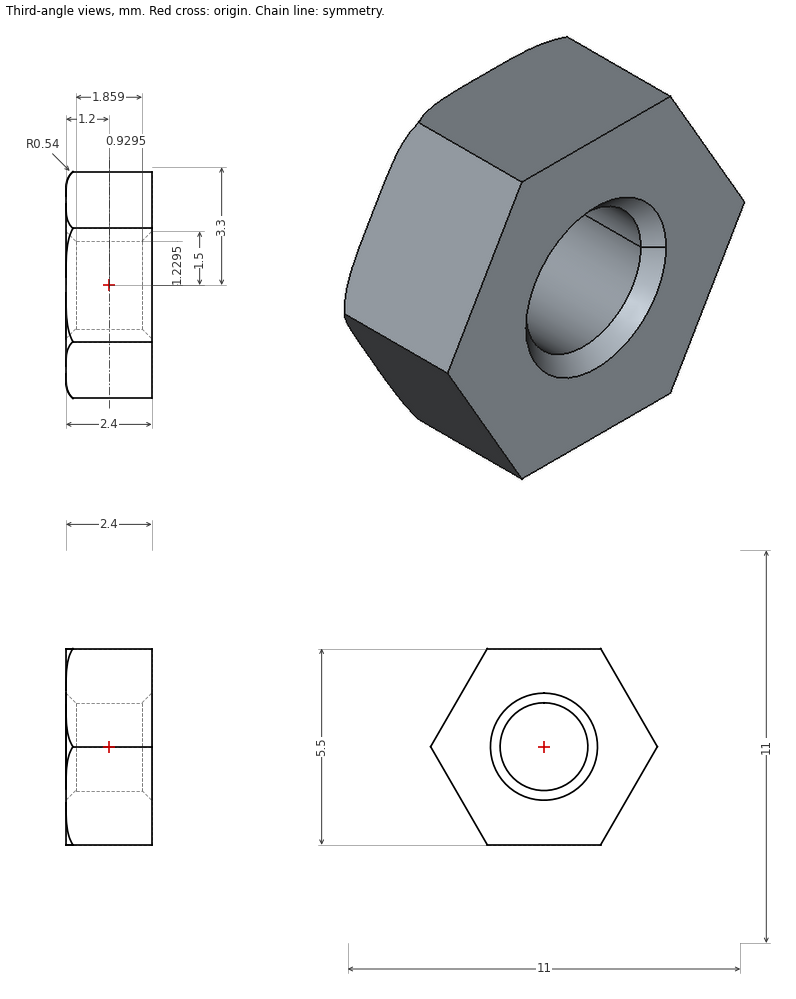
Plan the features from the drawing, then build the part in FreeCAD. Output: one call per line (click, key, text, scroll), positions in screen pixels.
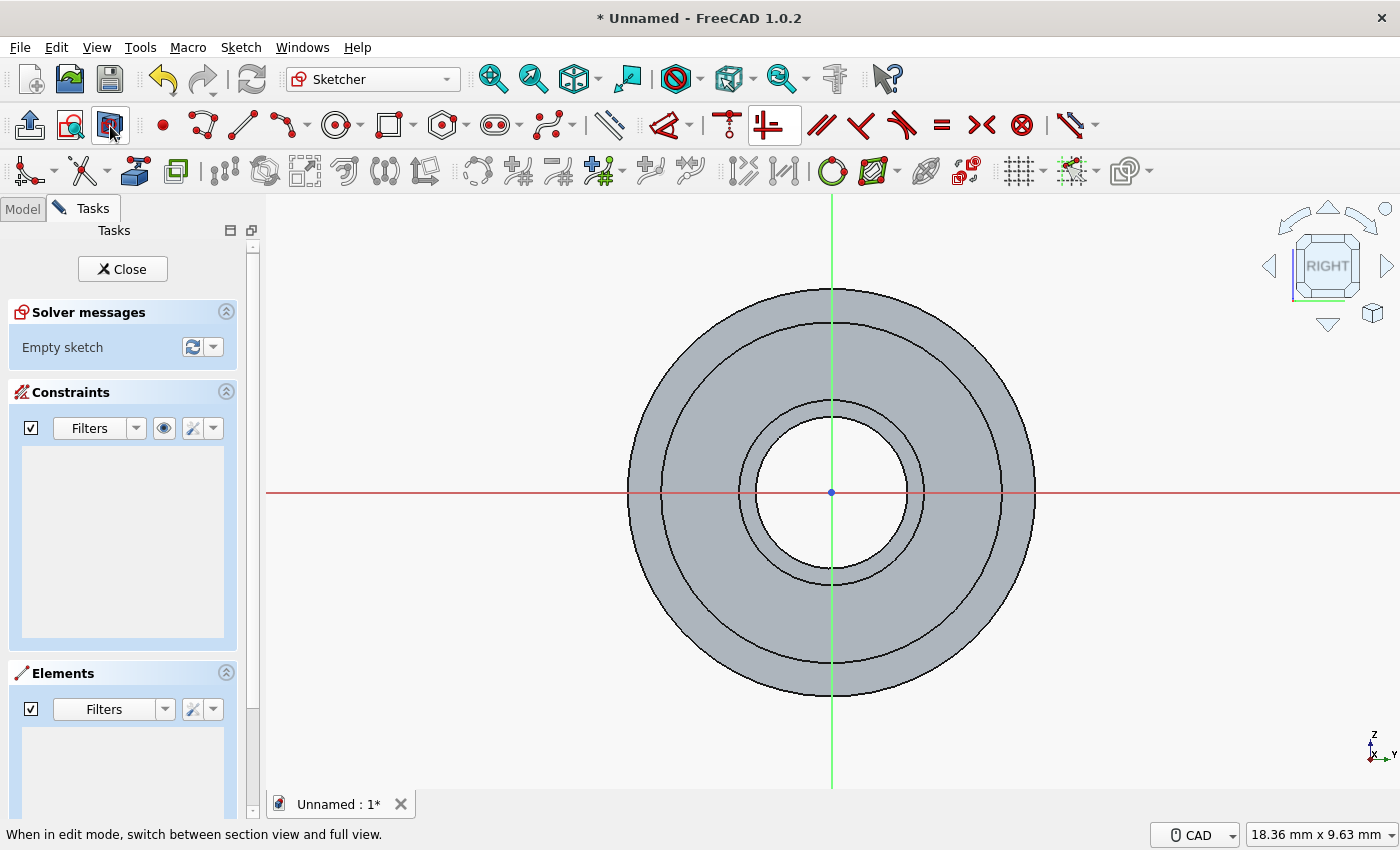
scroll(683, 490, down, 3)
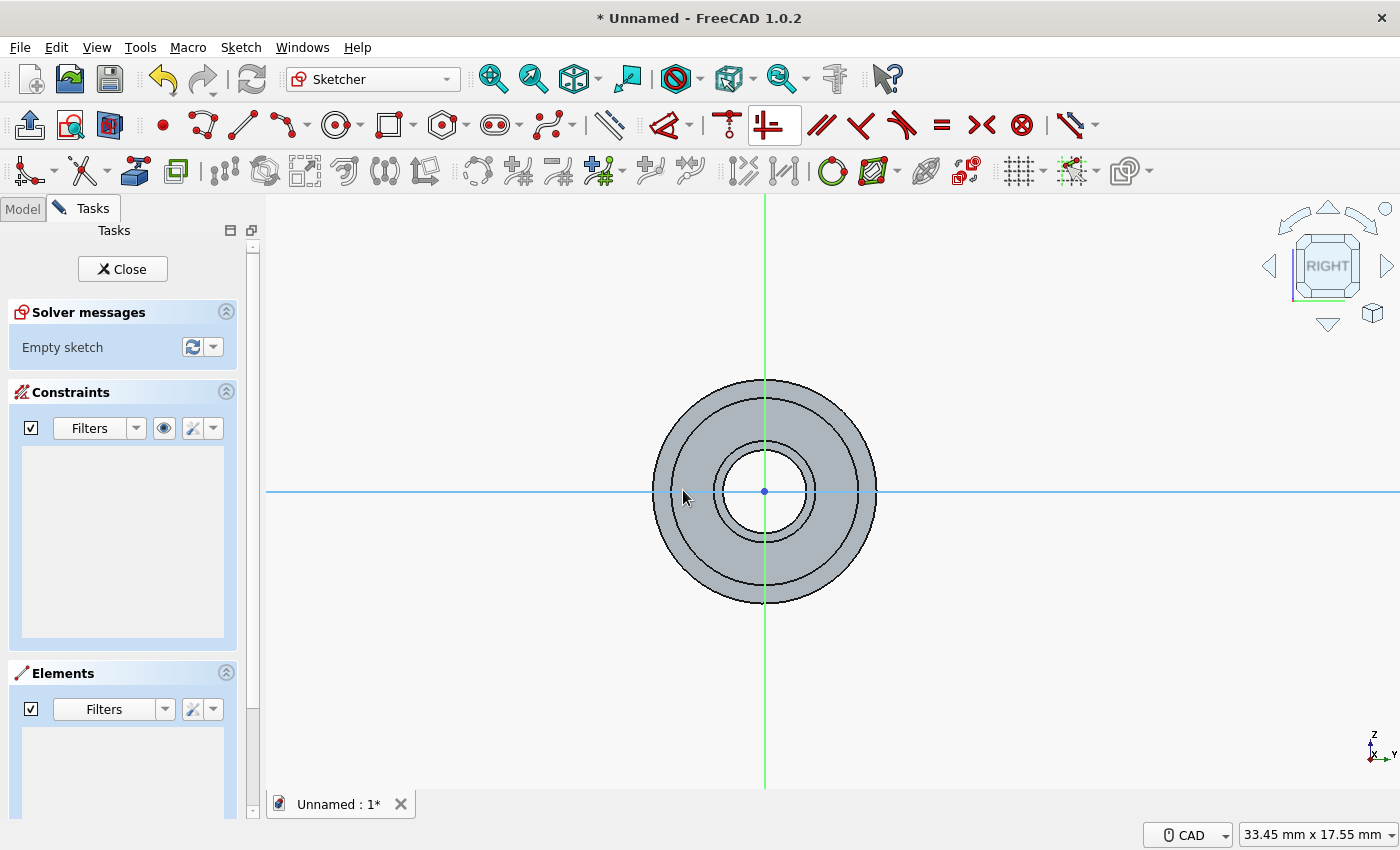
click(416, 126)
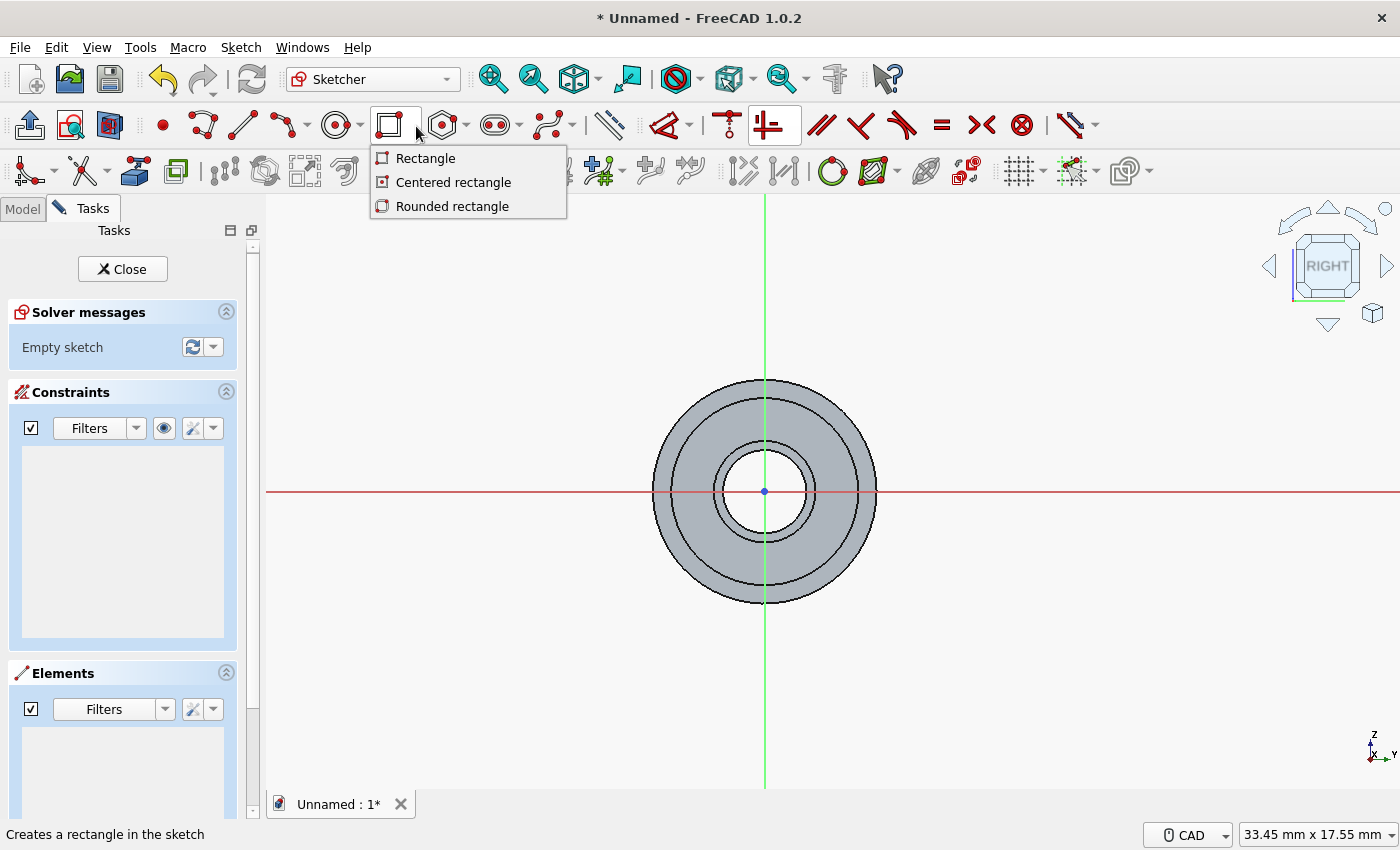
click(468, 182)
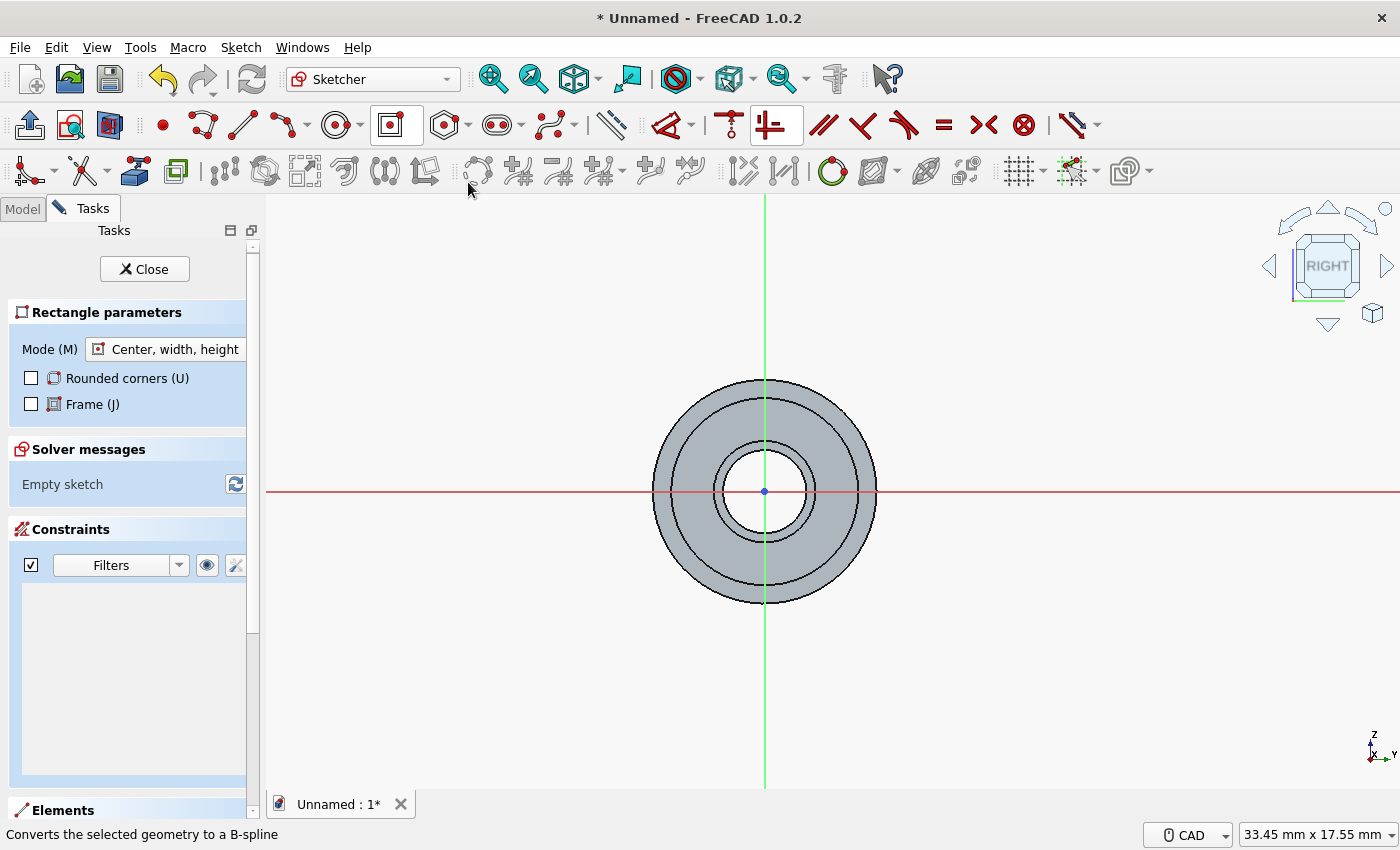
click(765, 492)
move(951, 305)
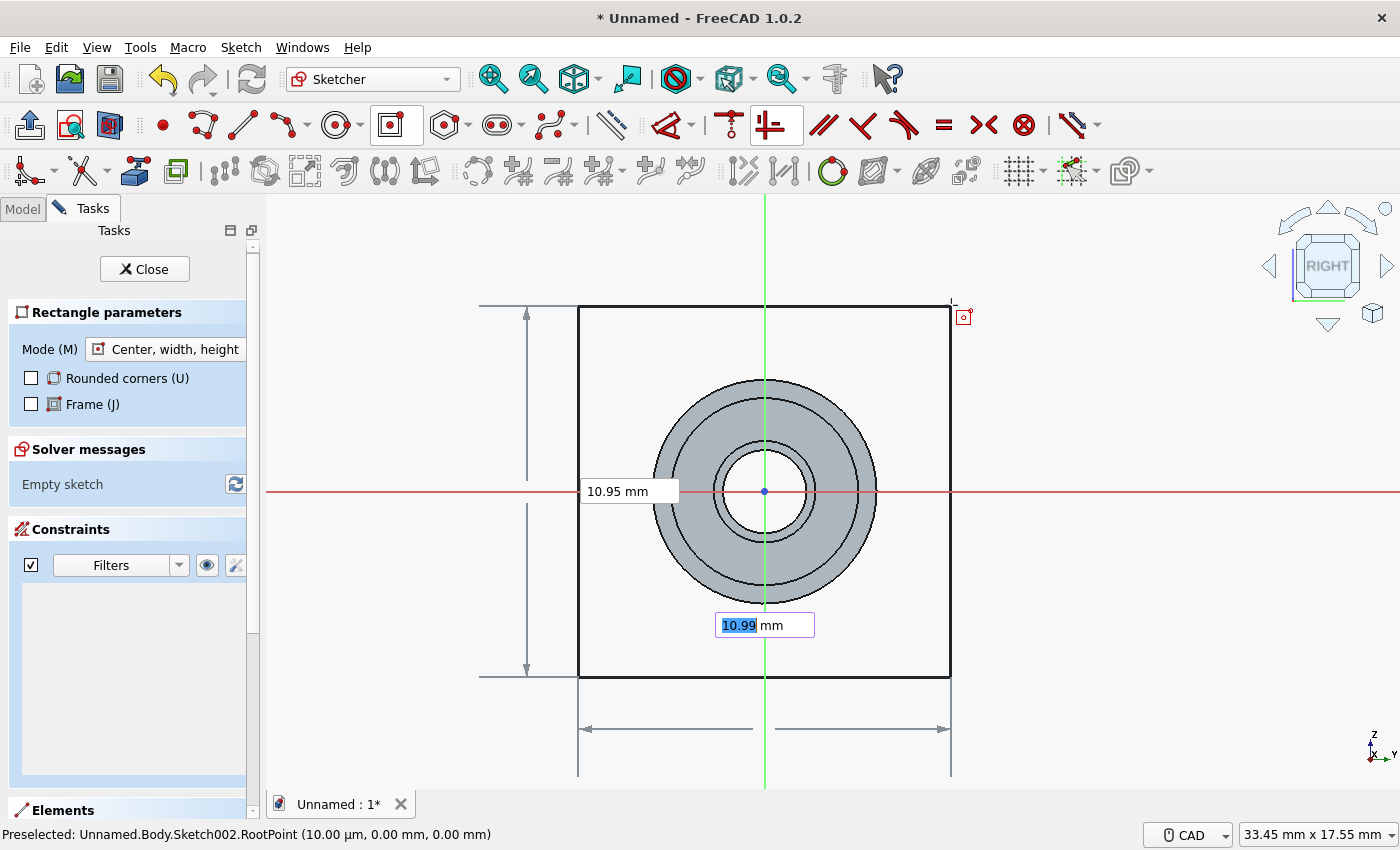
text(11)
key(Tab)
text(11)
key(Return)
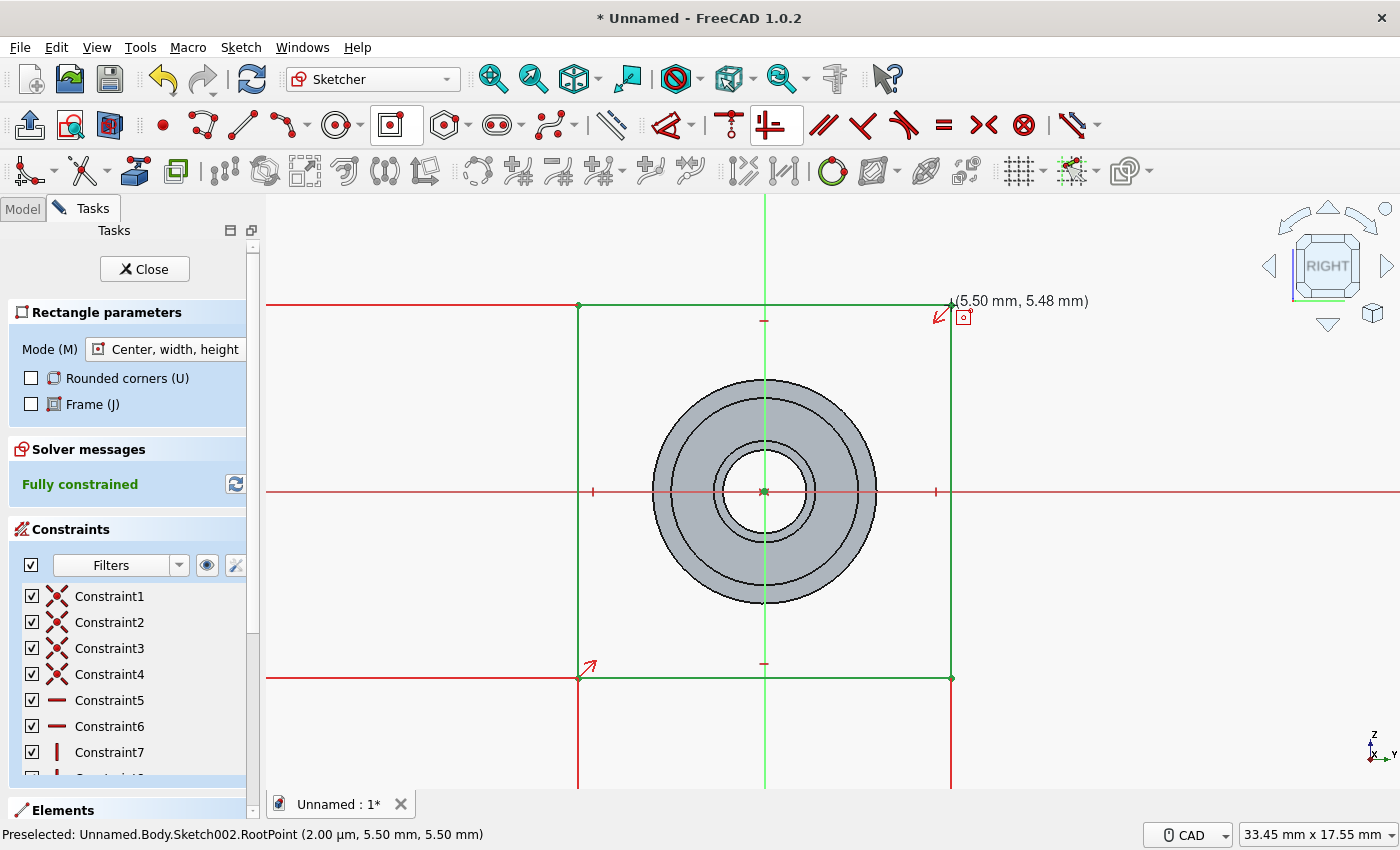
click(444, 126)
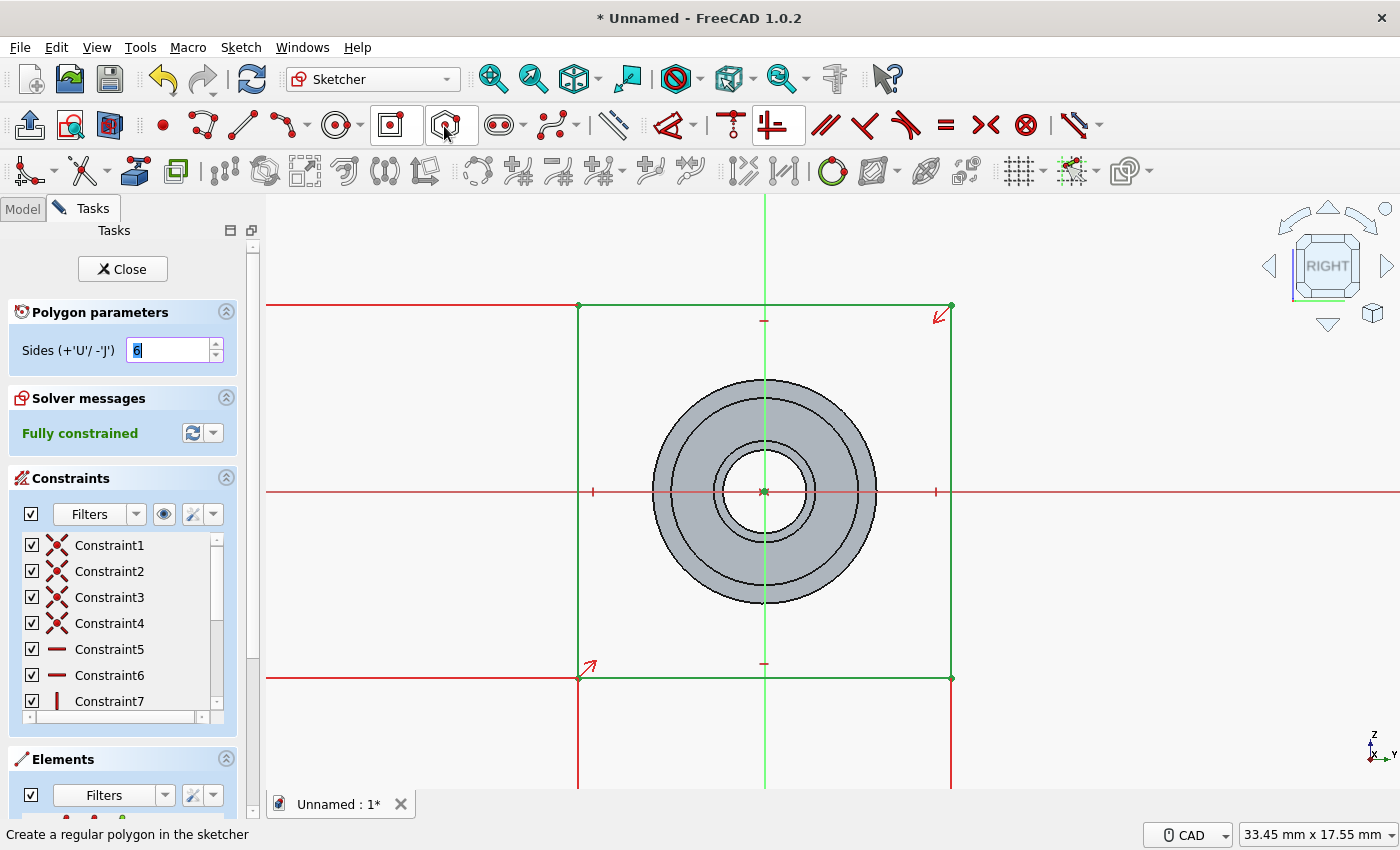
click(765, 492)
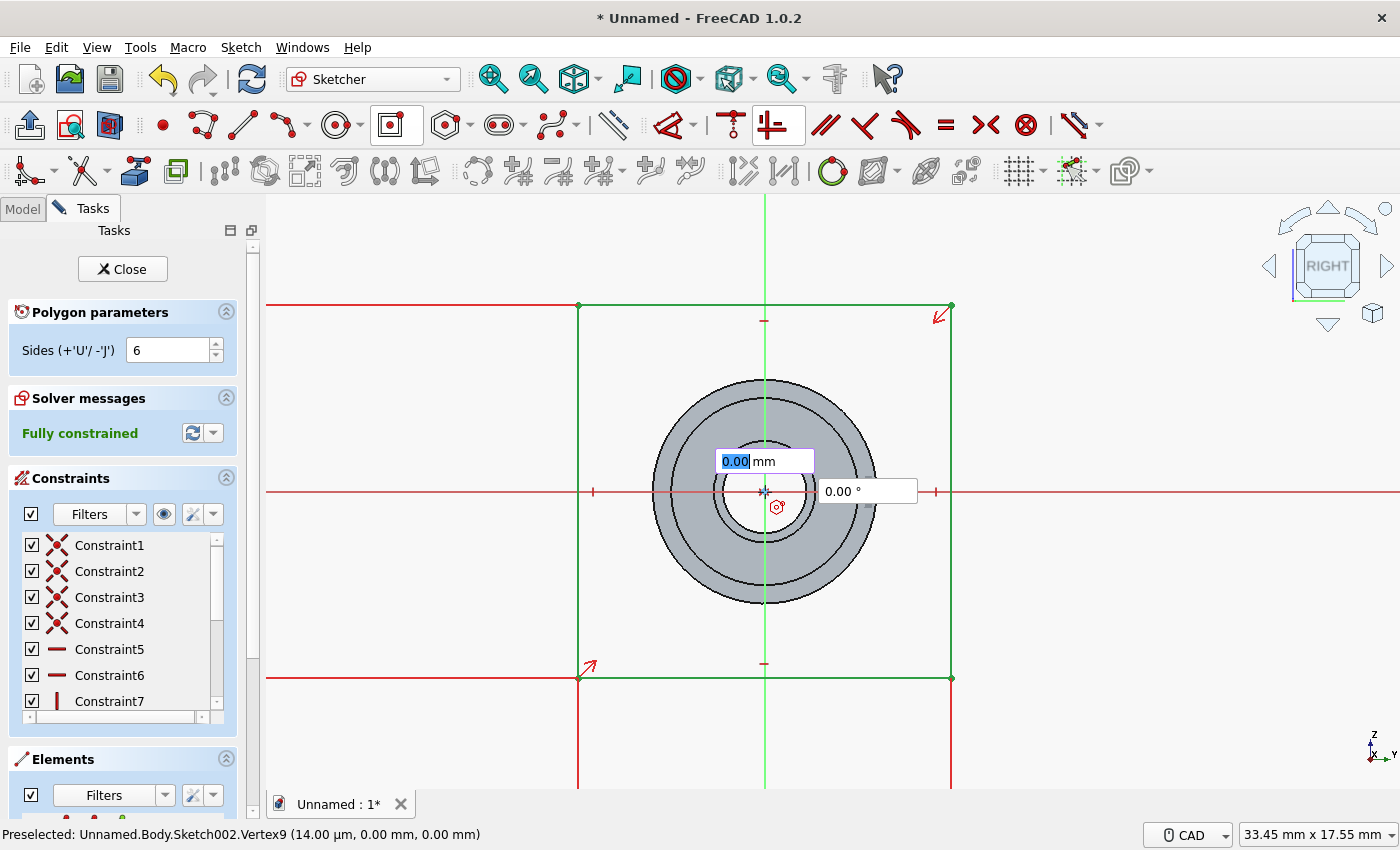
click(872, 492)
right_click(872, 492)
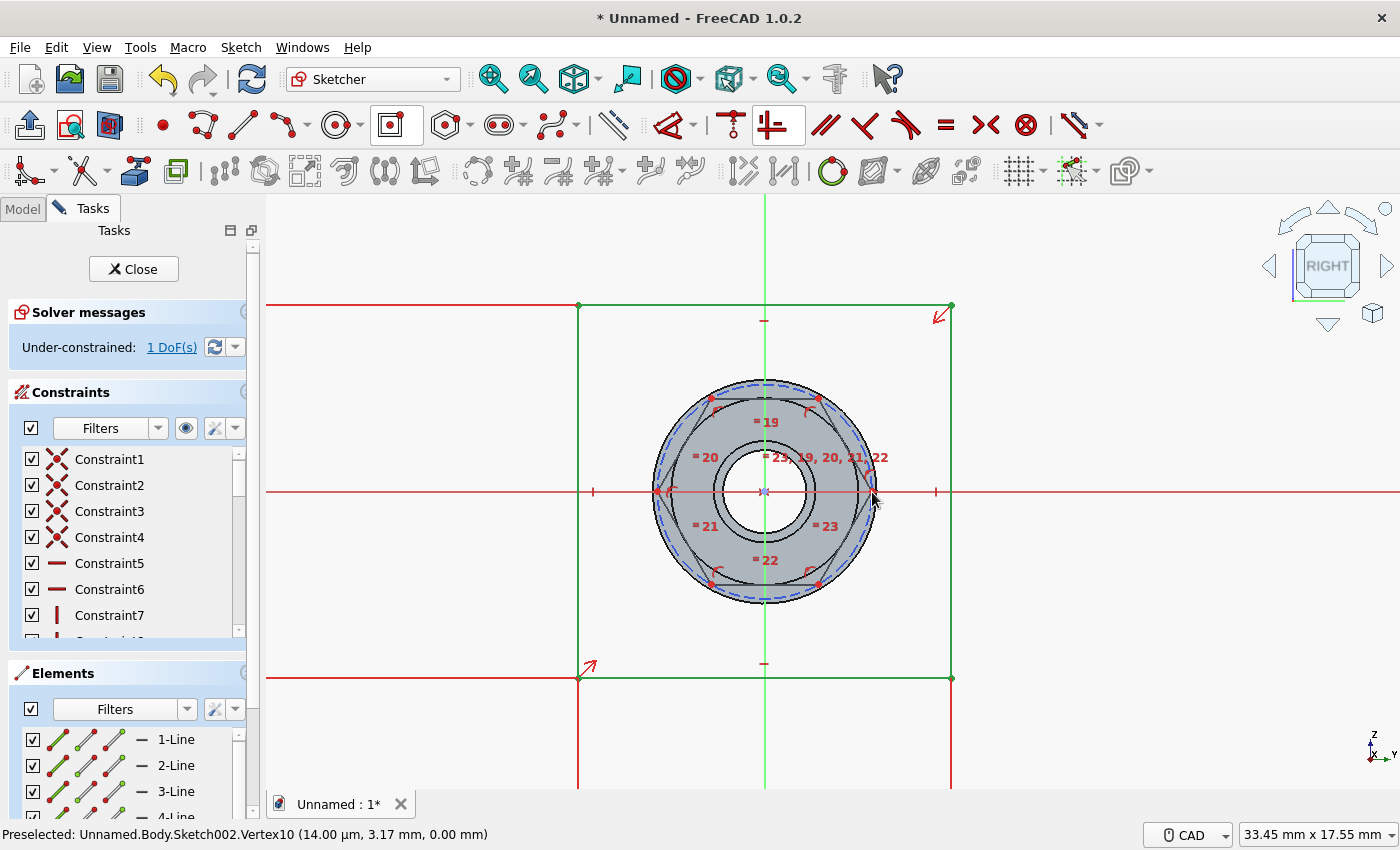
click(668, 126)